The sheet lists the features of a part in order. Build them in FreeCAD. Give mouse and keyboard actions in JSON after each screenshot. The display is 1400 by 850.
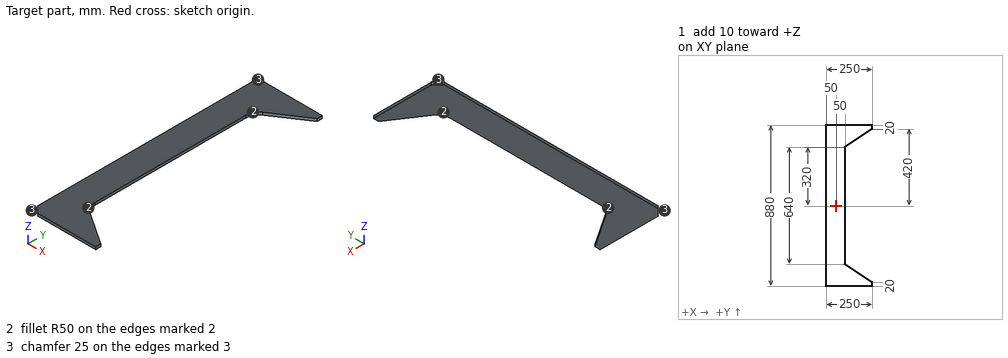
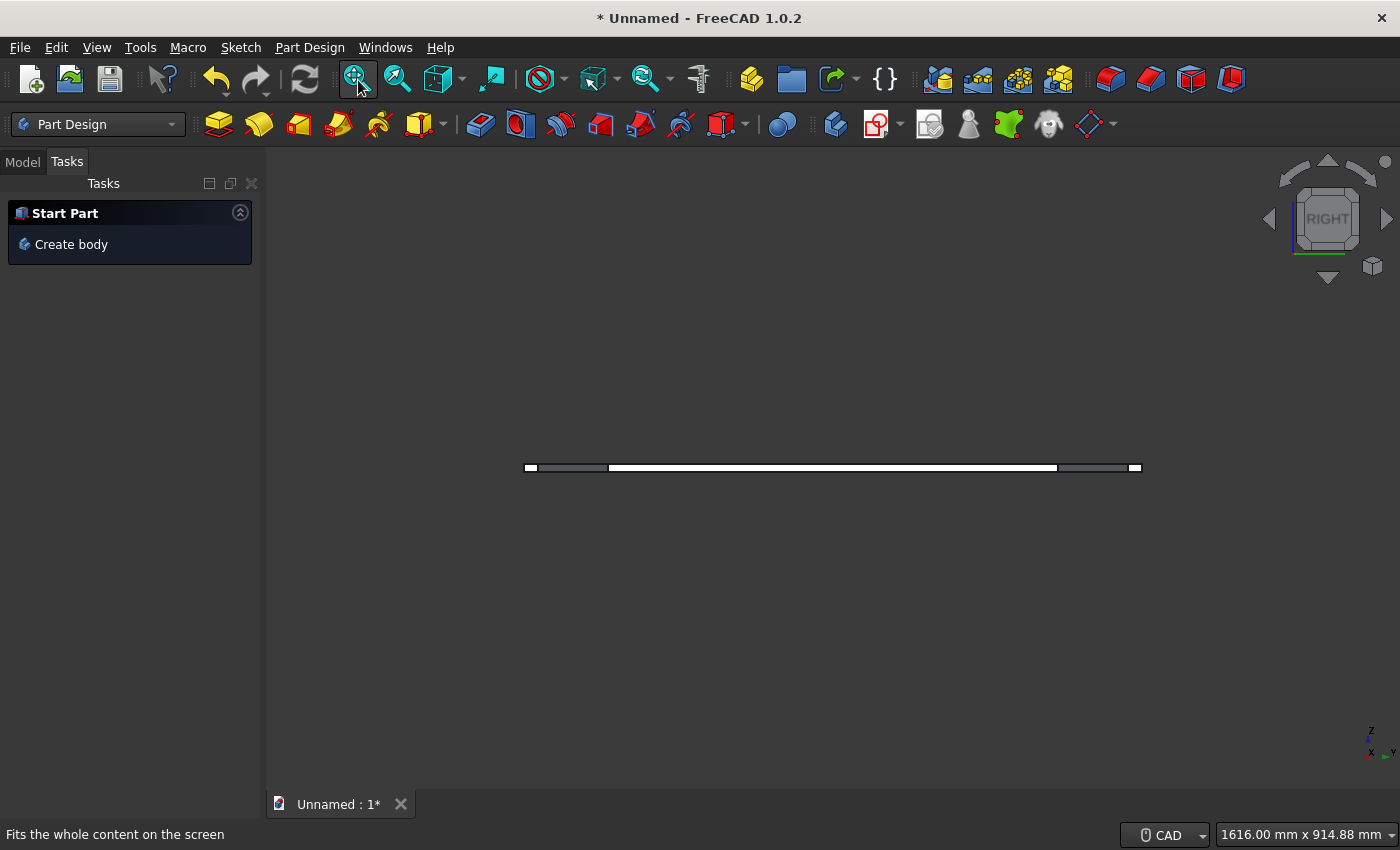
{"action": "key", "text": "5"}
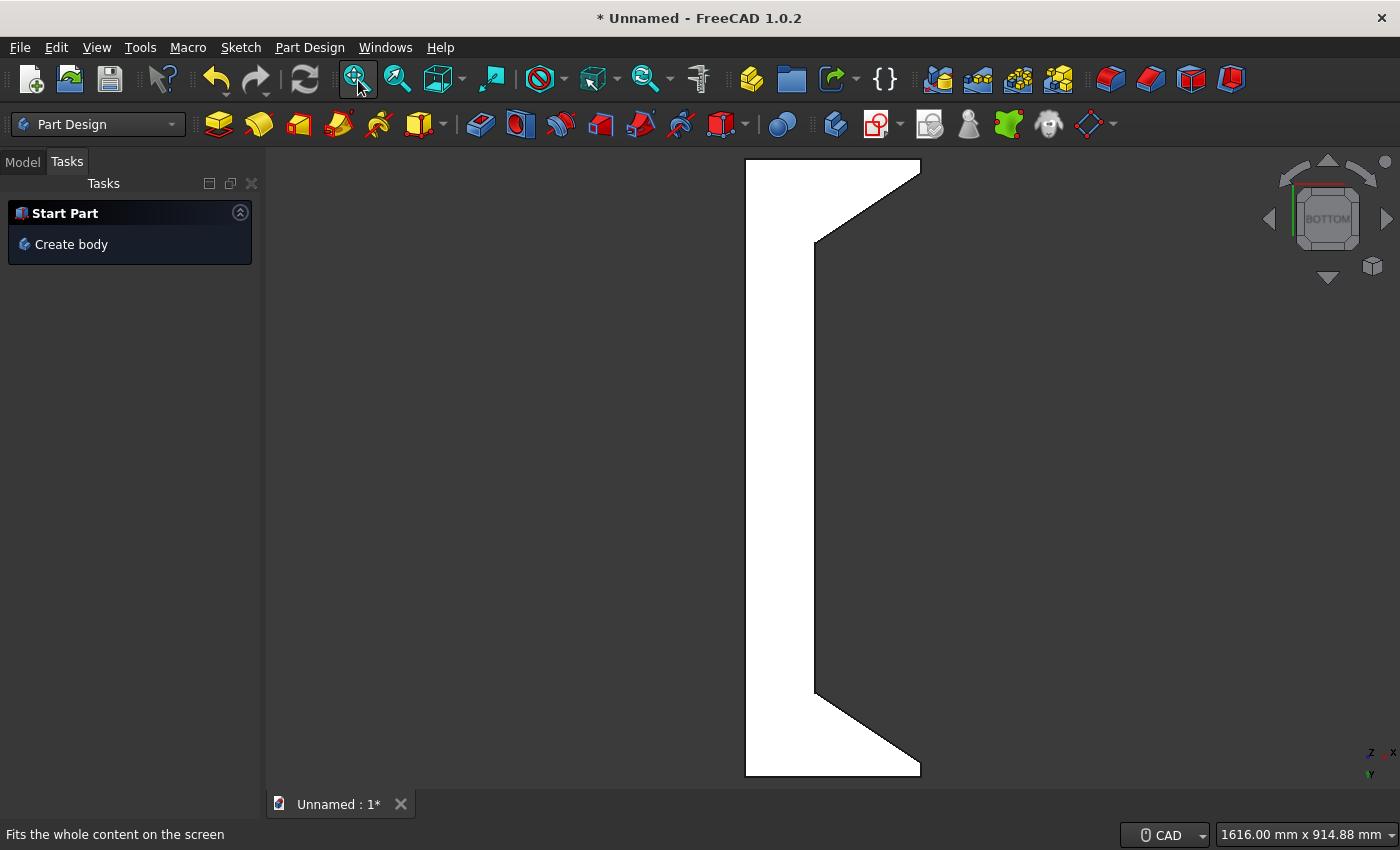
{"action": "scroll", "coordinate": [815, 692], "scroll_direction": "up", "scroll_amount": 9}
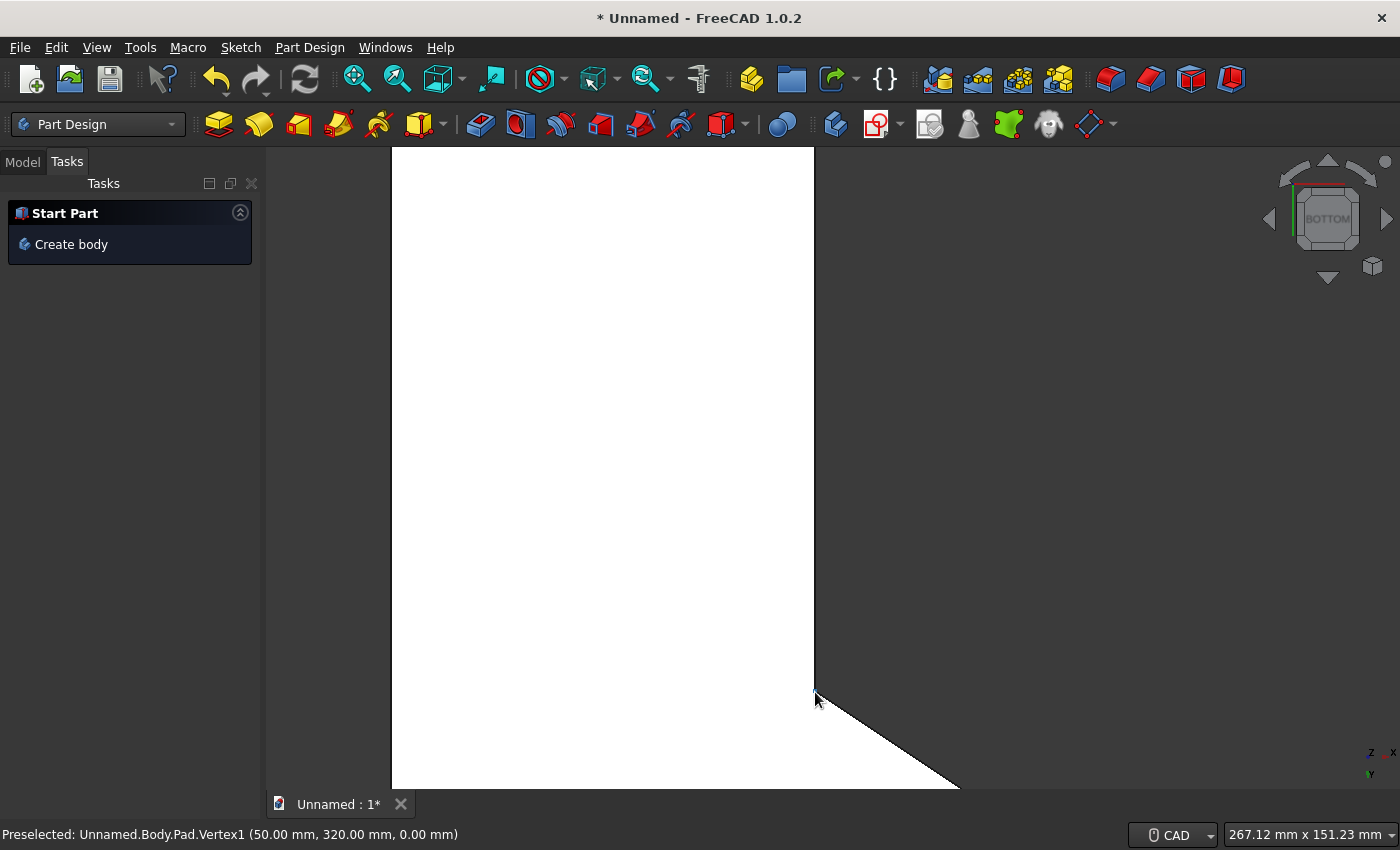
{"action": "key", "text": "v f"}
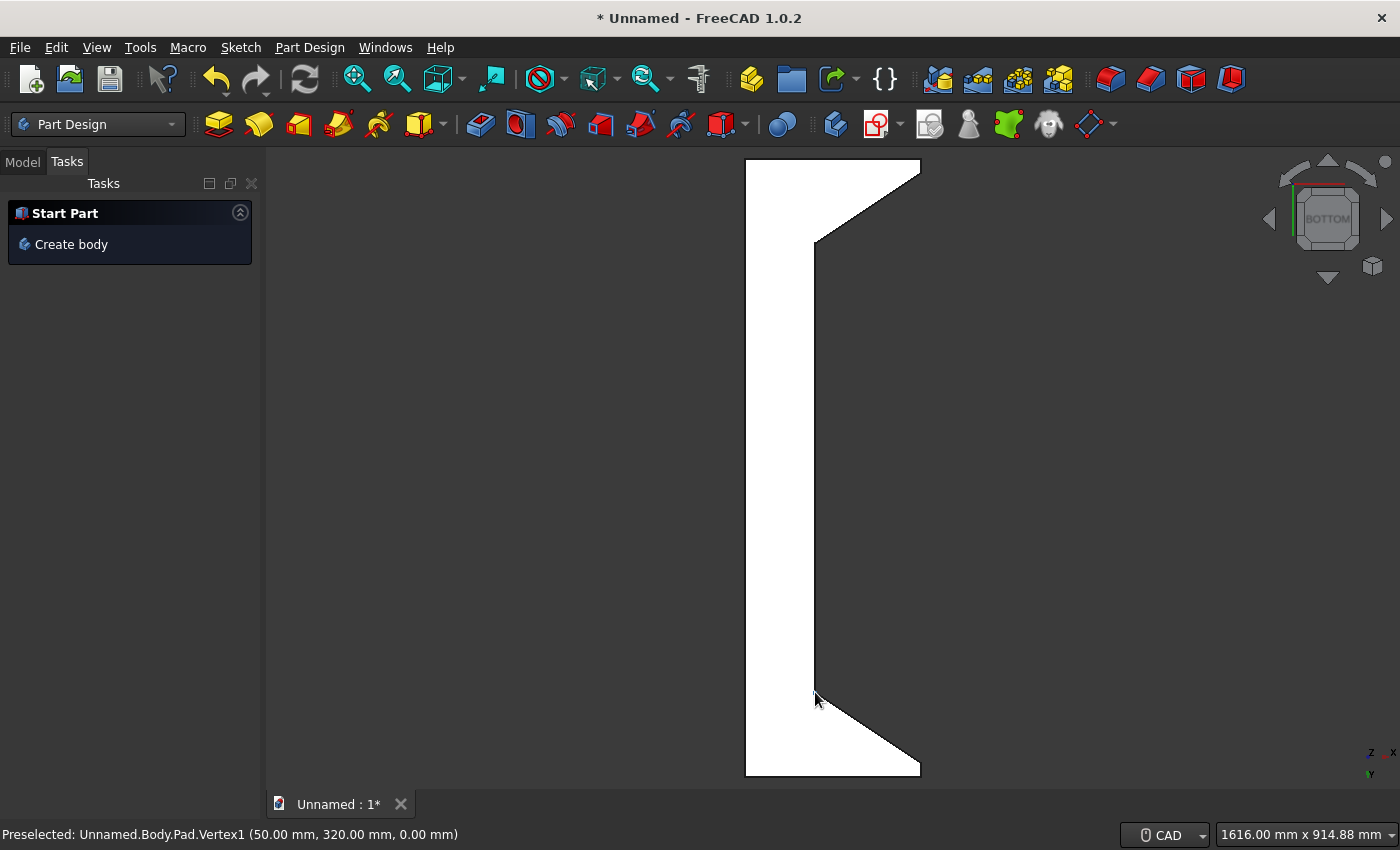
{"action": "key", "text": "4"}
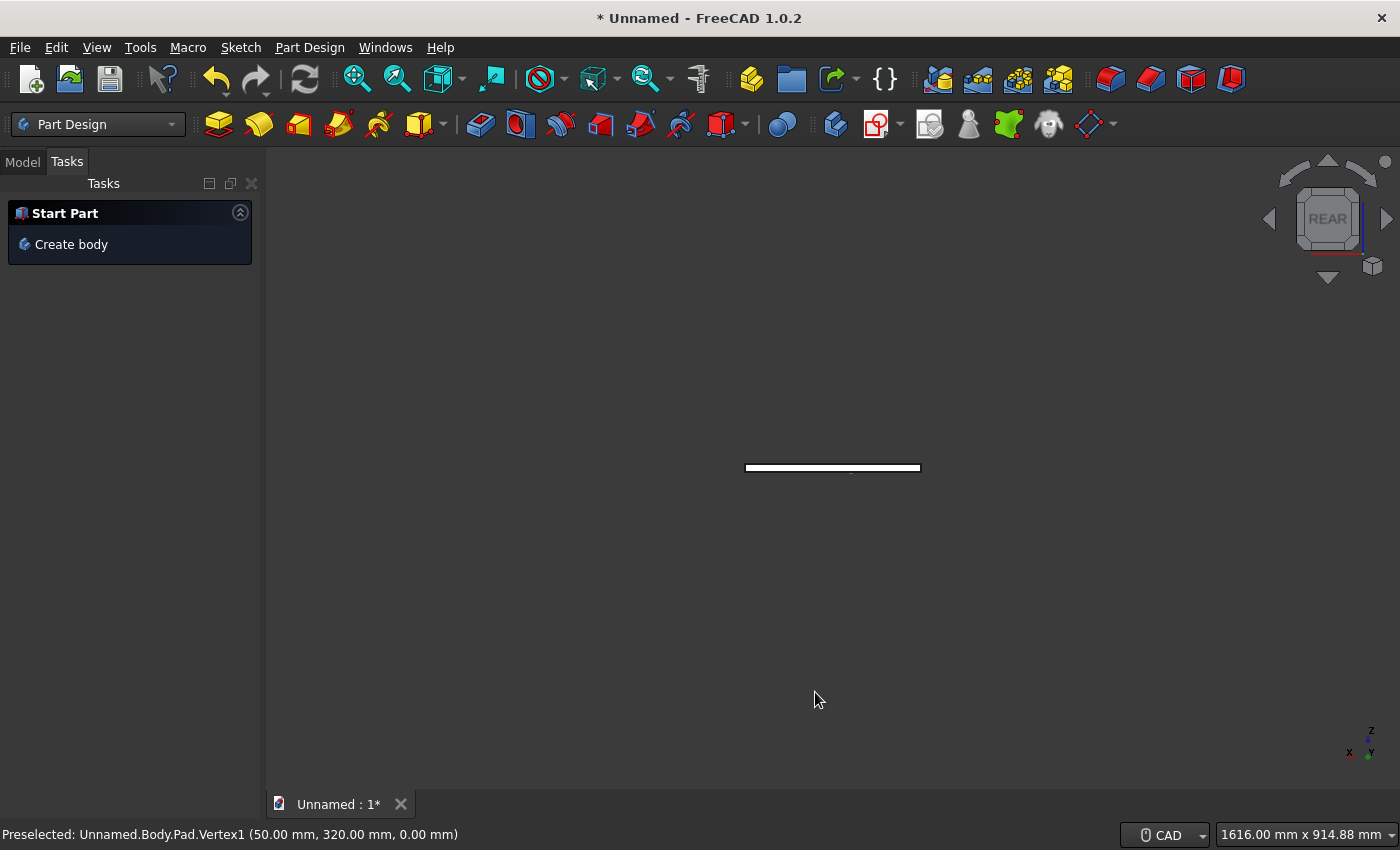
{"action": "left_click", "coordinate": [358, 80]}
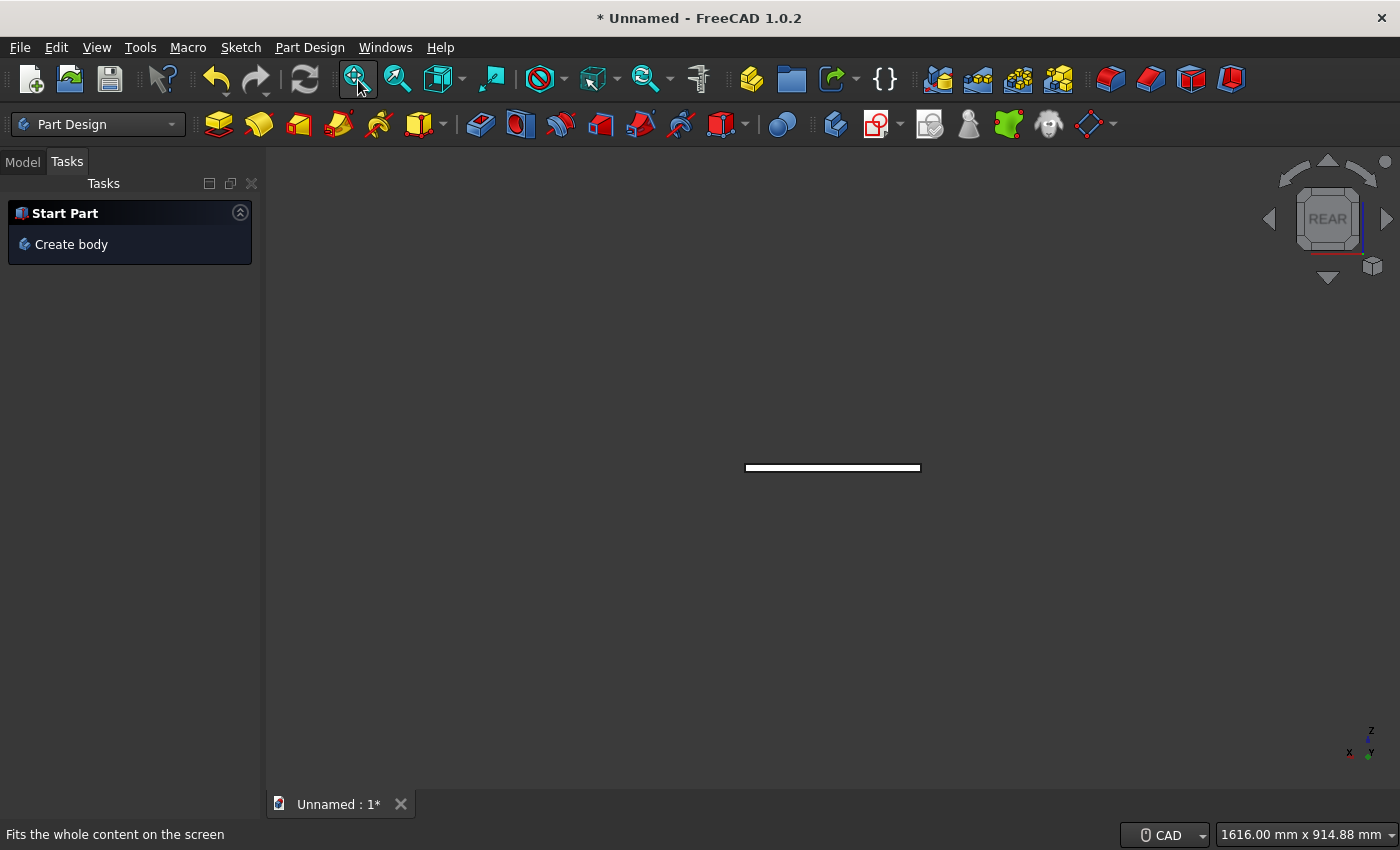
{"action": "scroll", "coordinate": [851, 467], "scroll_direction": "up", "scroll_amount": 9}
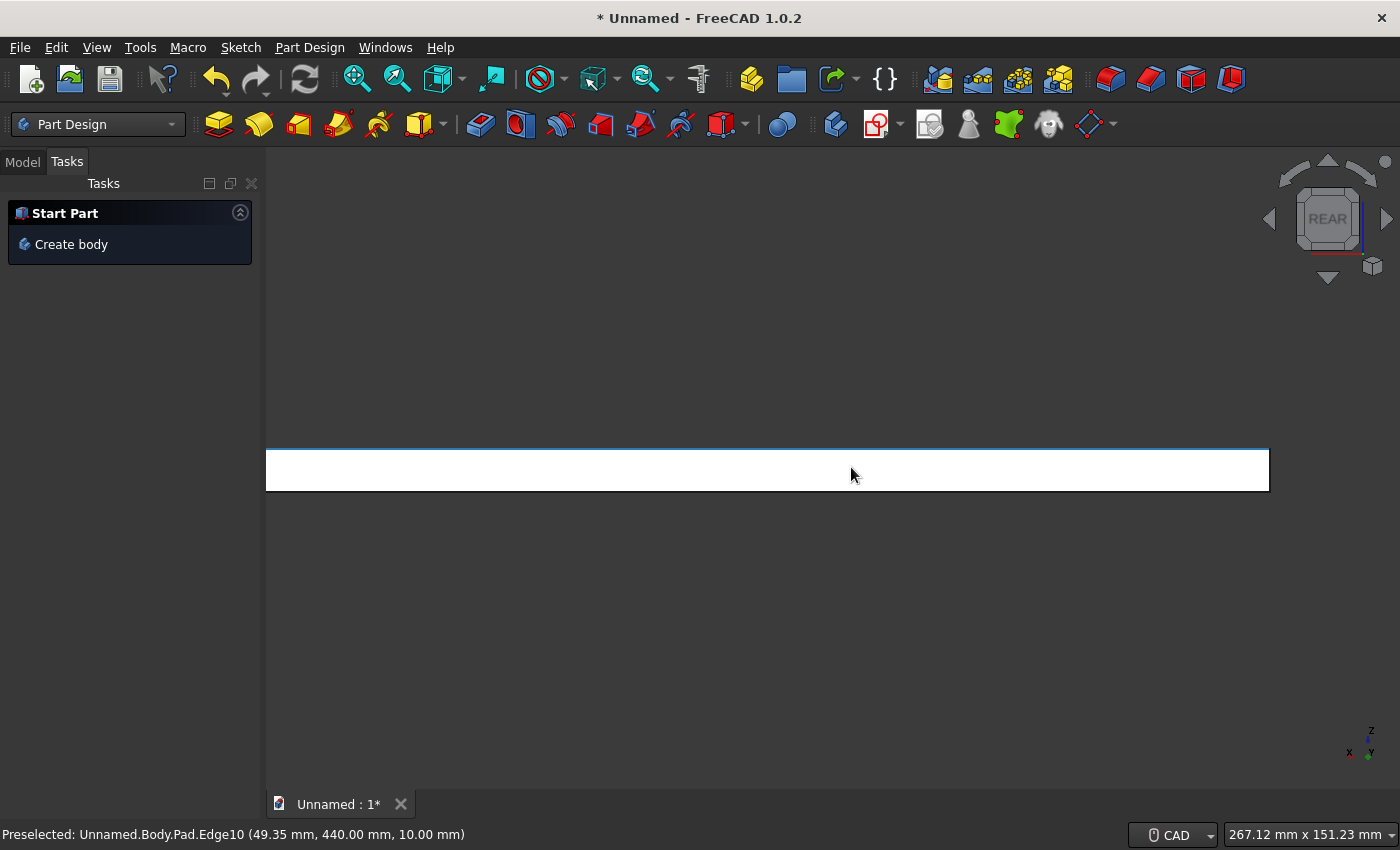
{"action": "key", "text": "v f"}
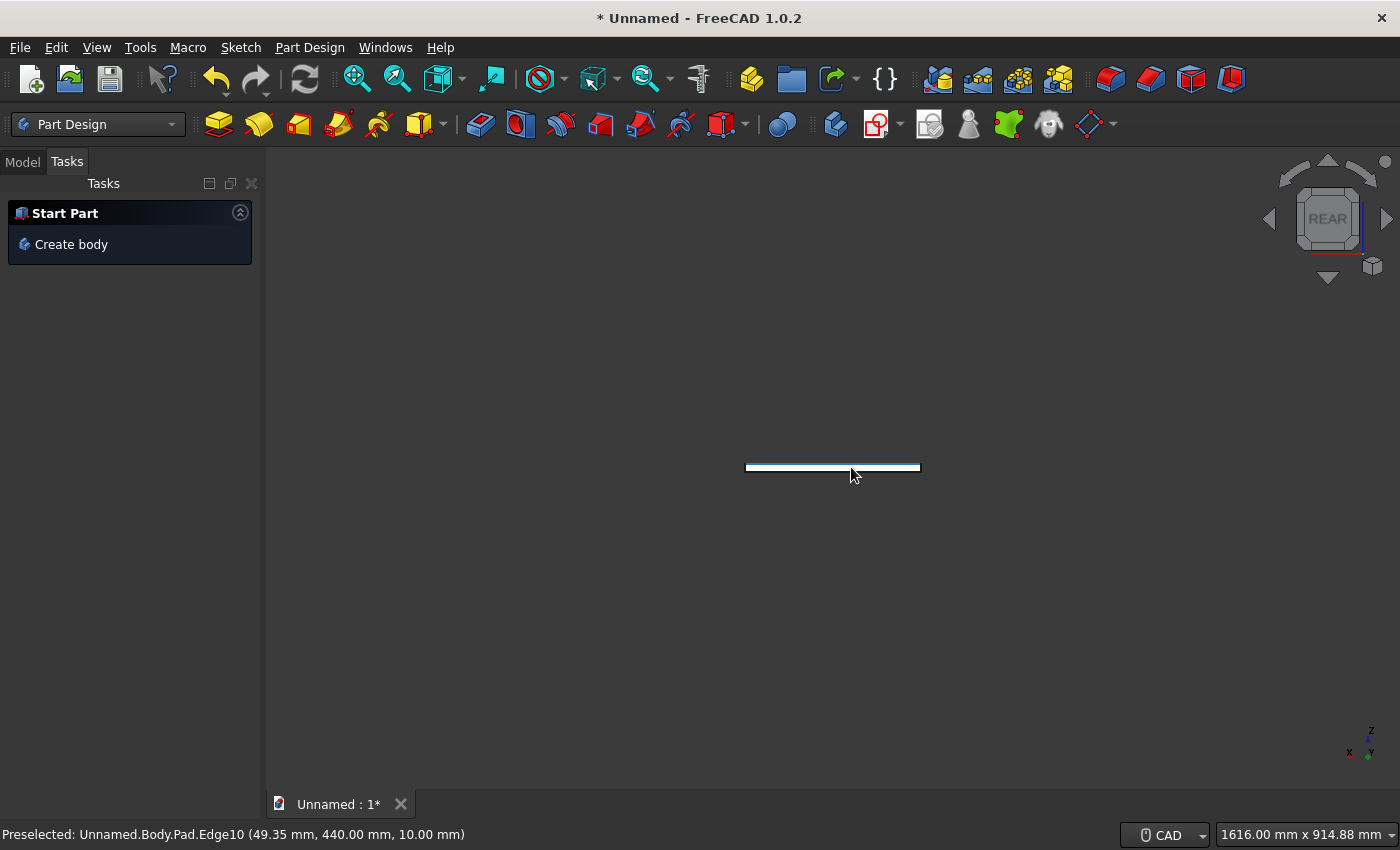
{"action": "key", "text": "6"}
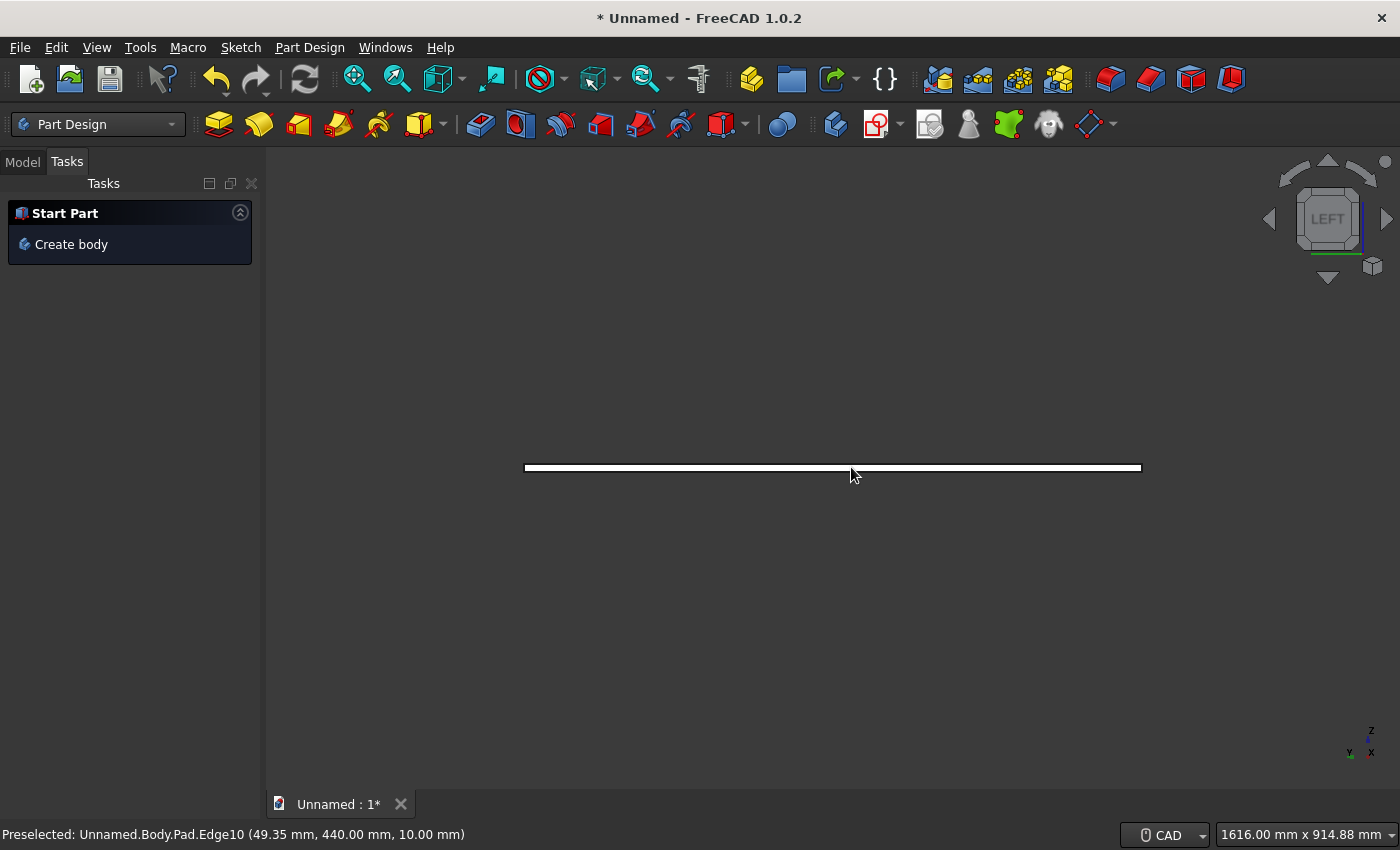
{"action": "scroll", "coordinate": [608, 467], "scroll_direction": "up", "scroll_amount": 9}